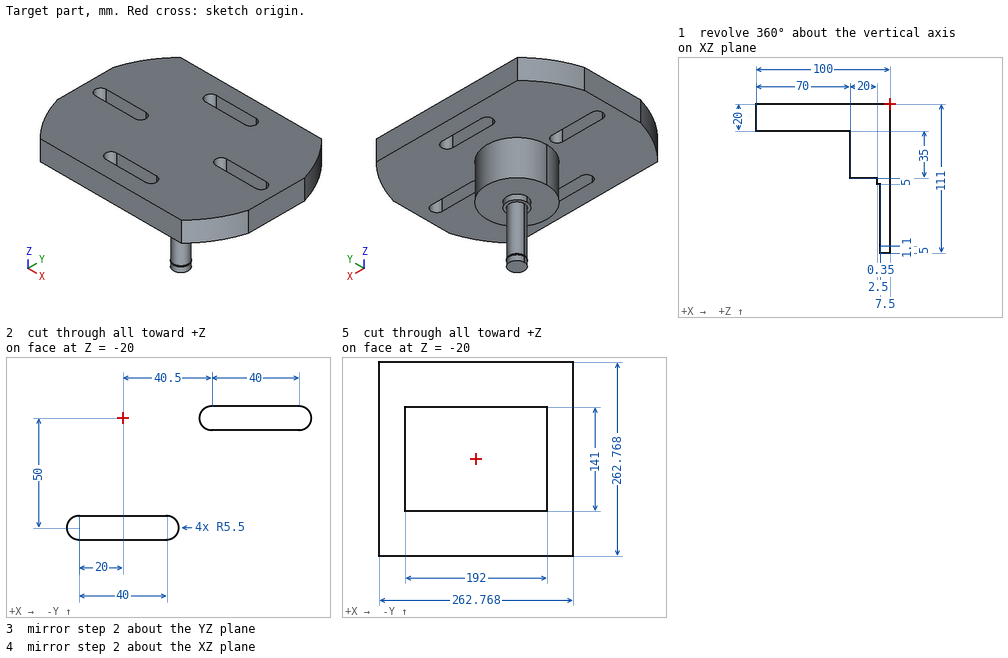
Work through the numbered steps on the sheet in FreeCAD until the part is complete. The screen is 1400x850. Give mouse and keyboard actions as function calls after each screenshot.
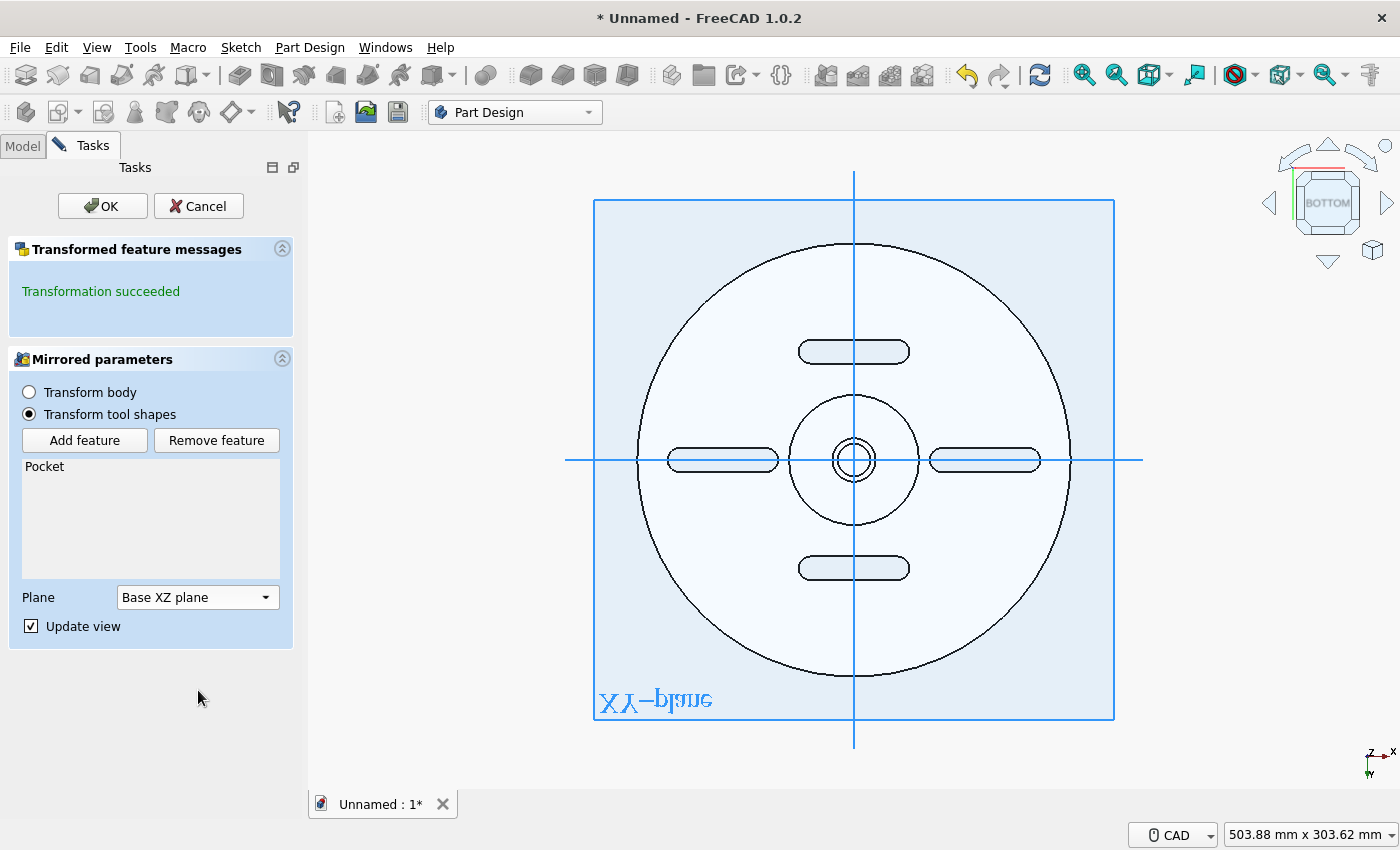
click(103, 206)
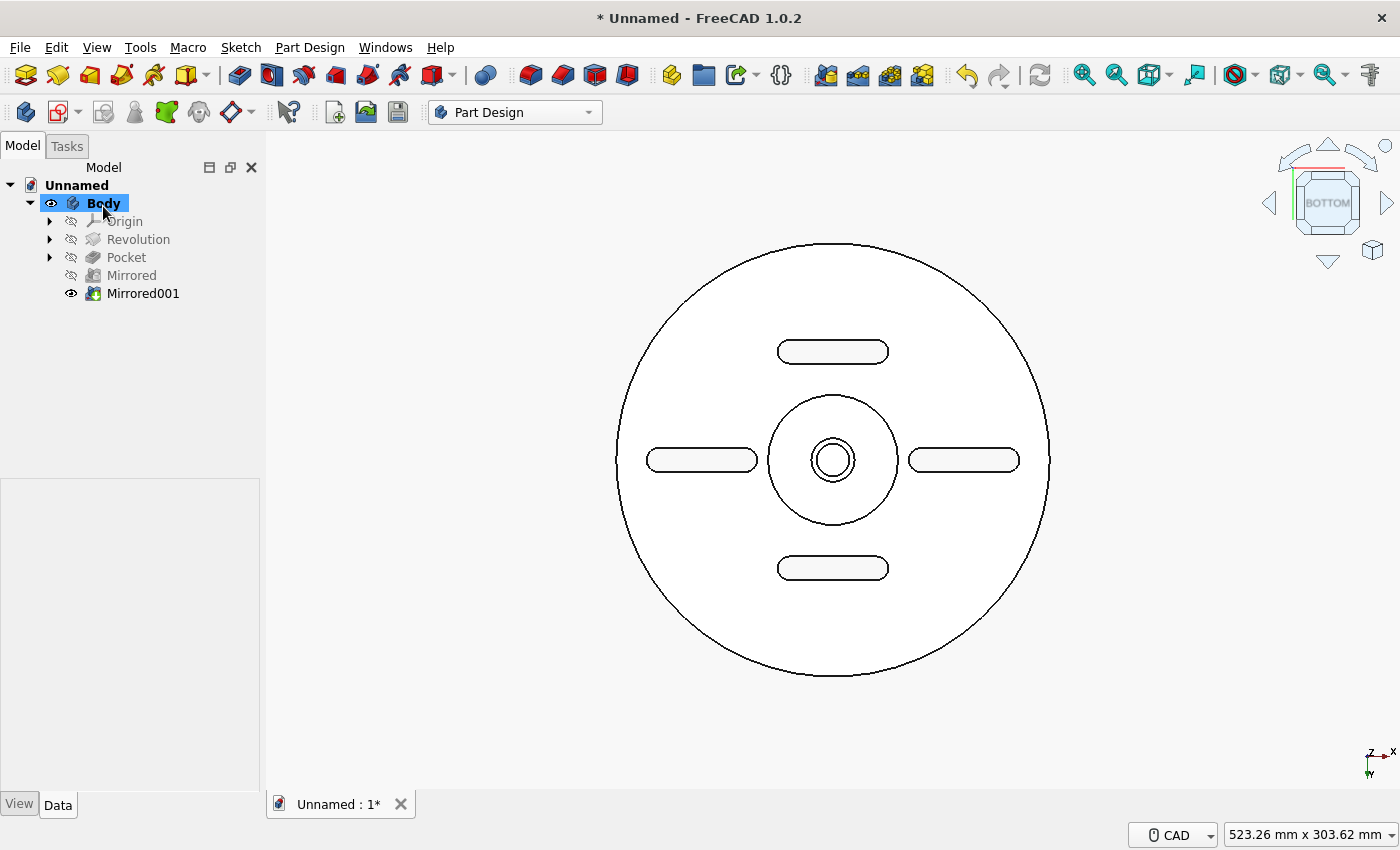
click(709, 397)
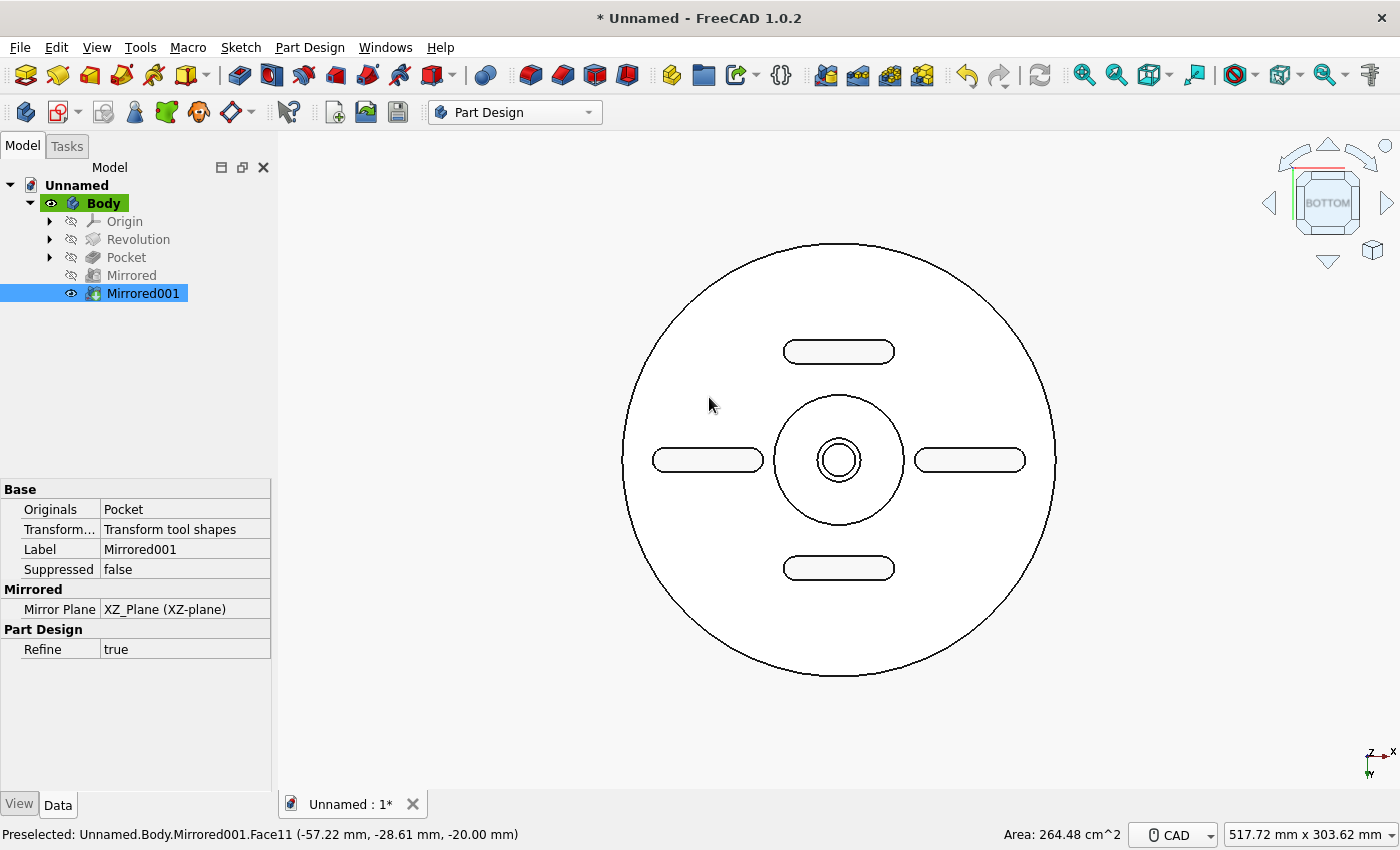
click(58, 112)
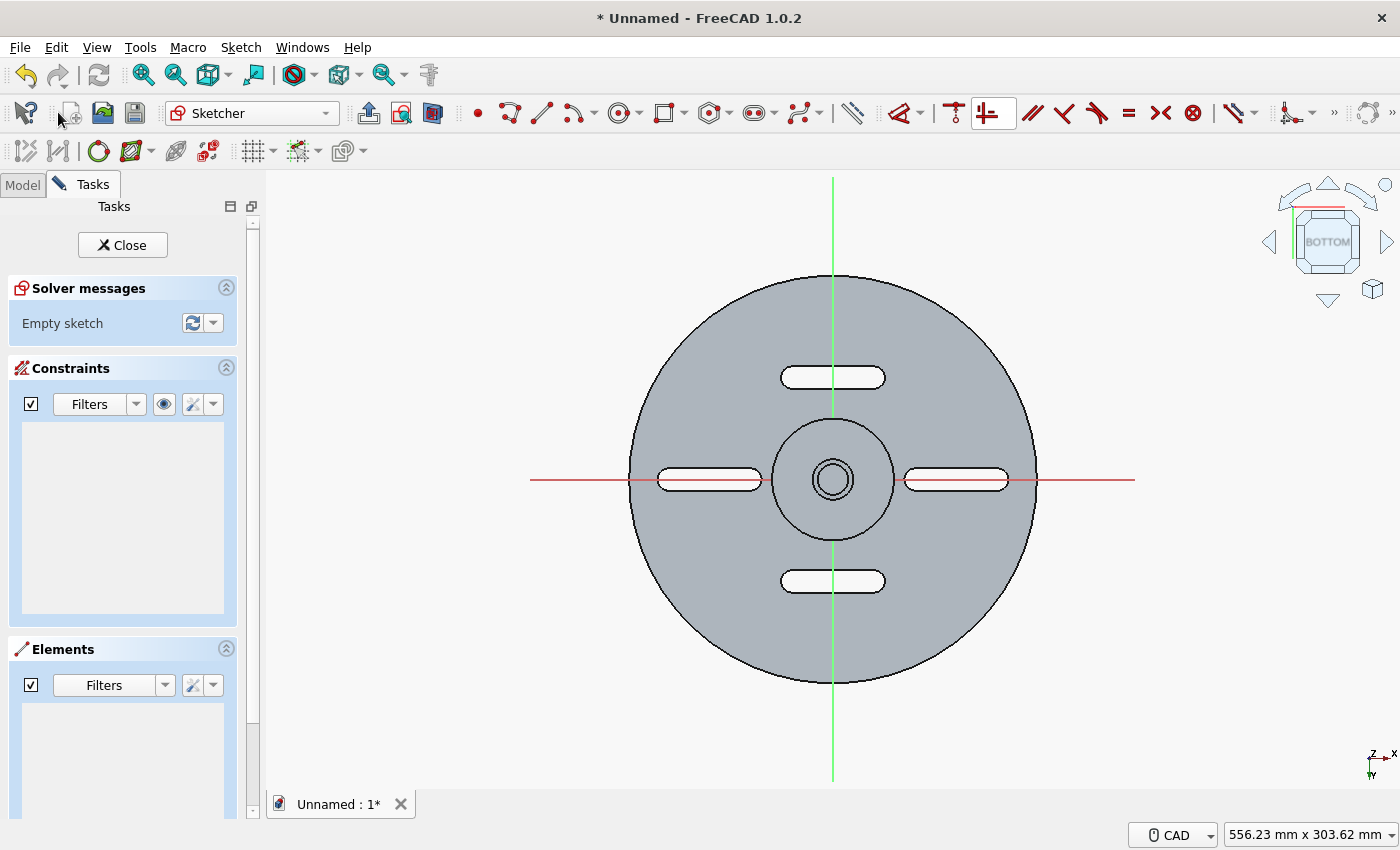
scroll(455, 479, down, 1)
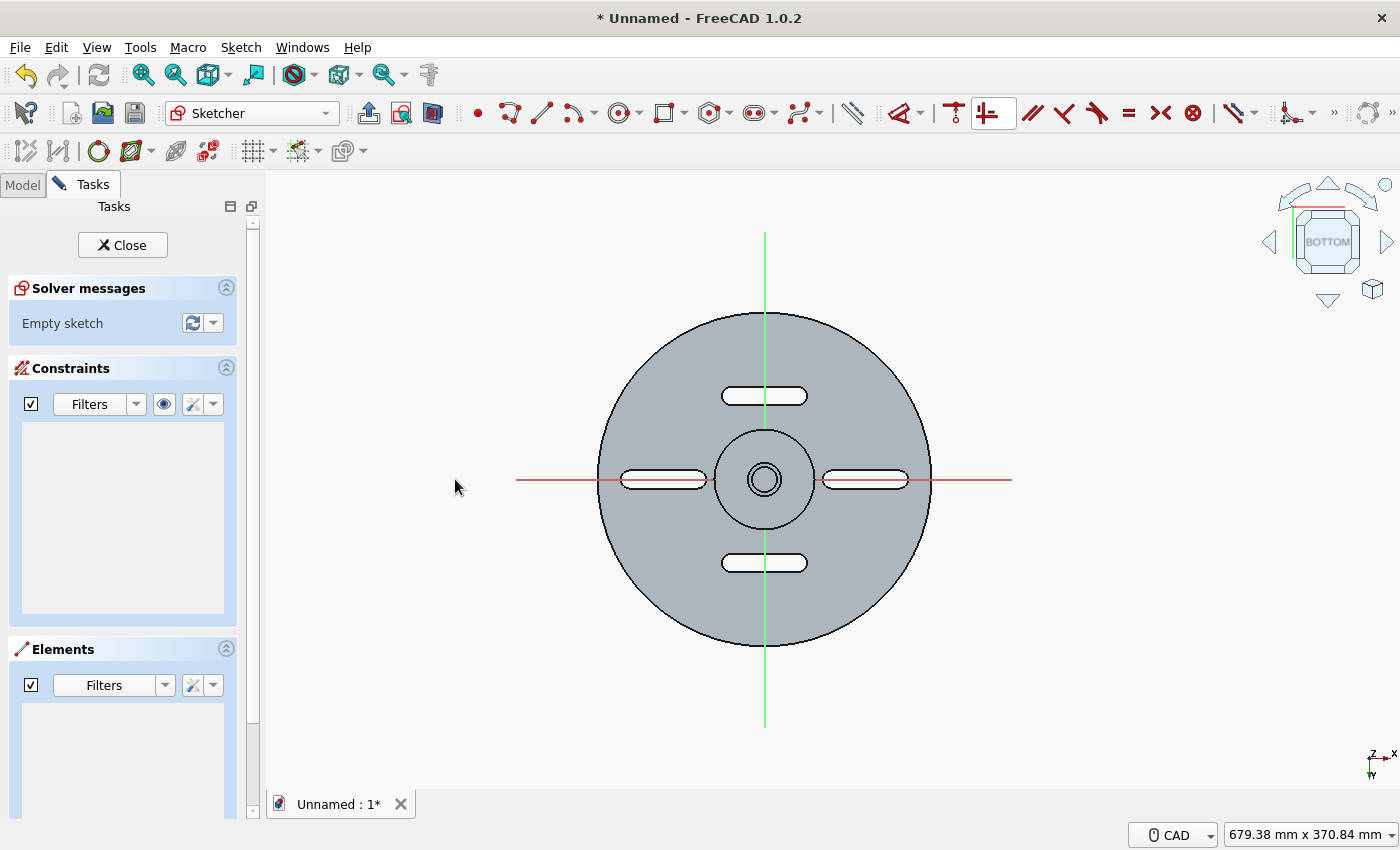
click(686, 114)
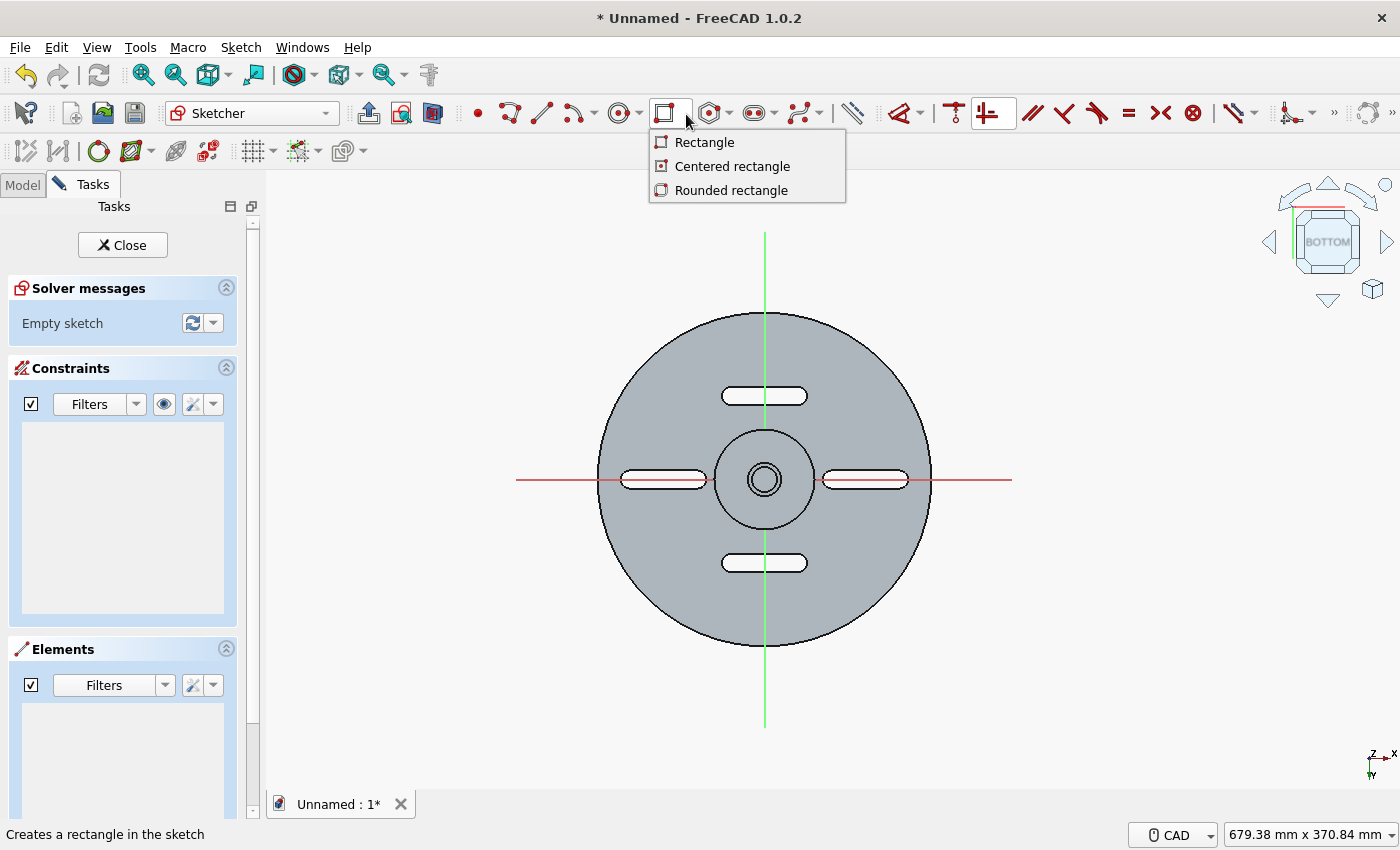
click(748, 166)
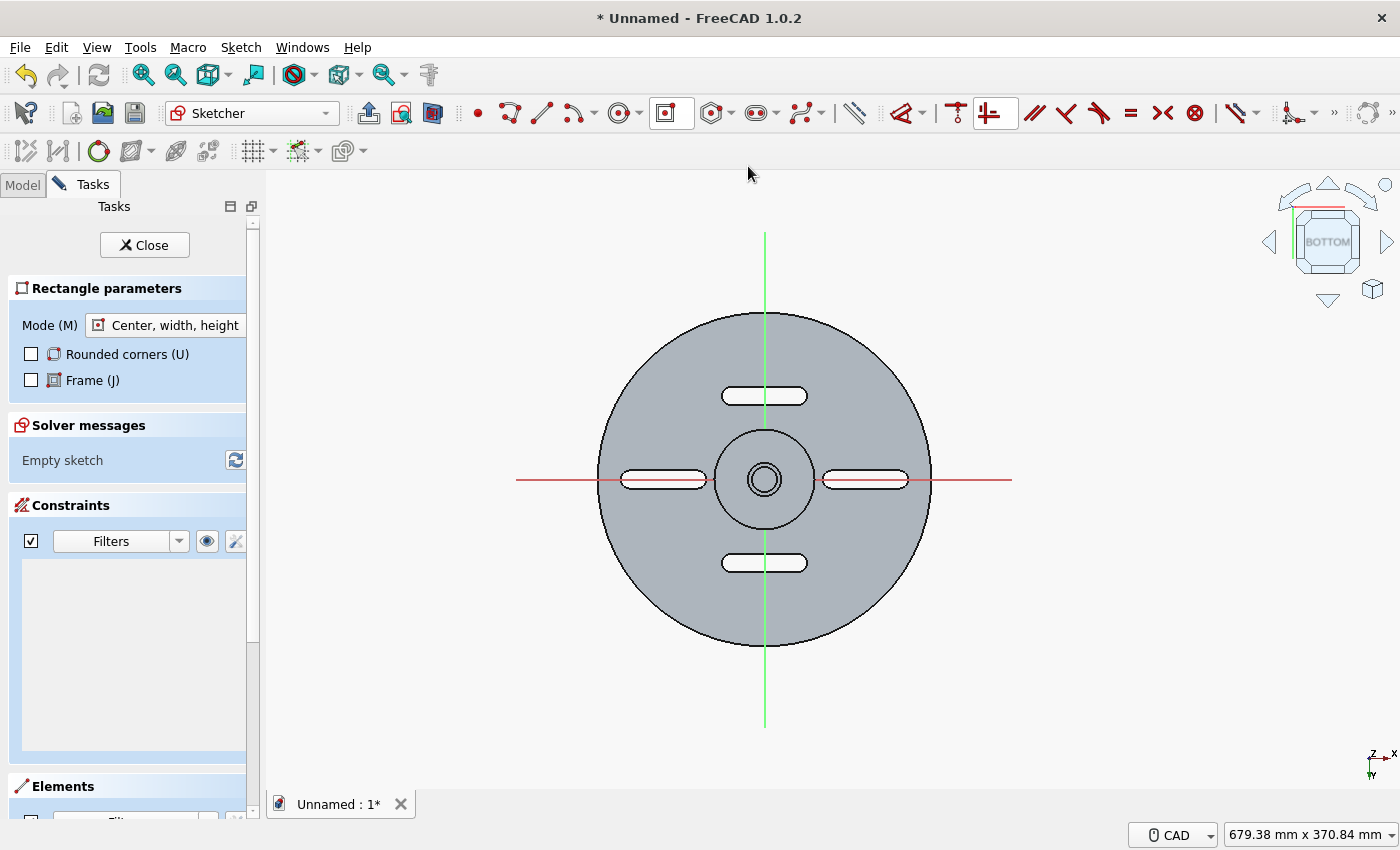
click(765, 480)
click(984, 260)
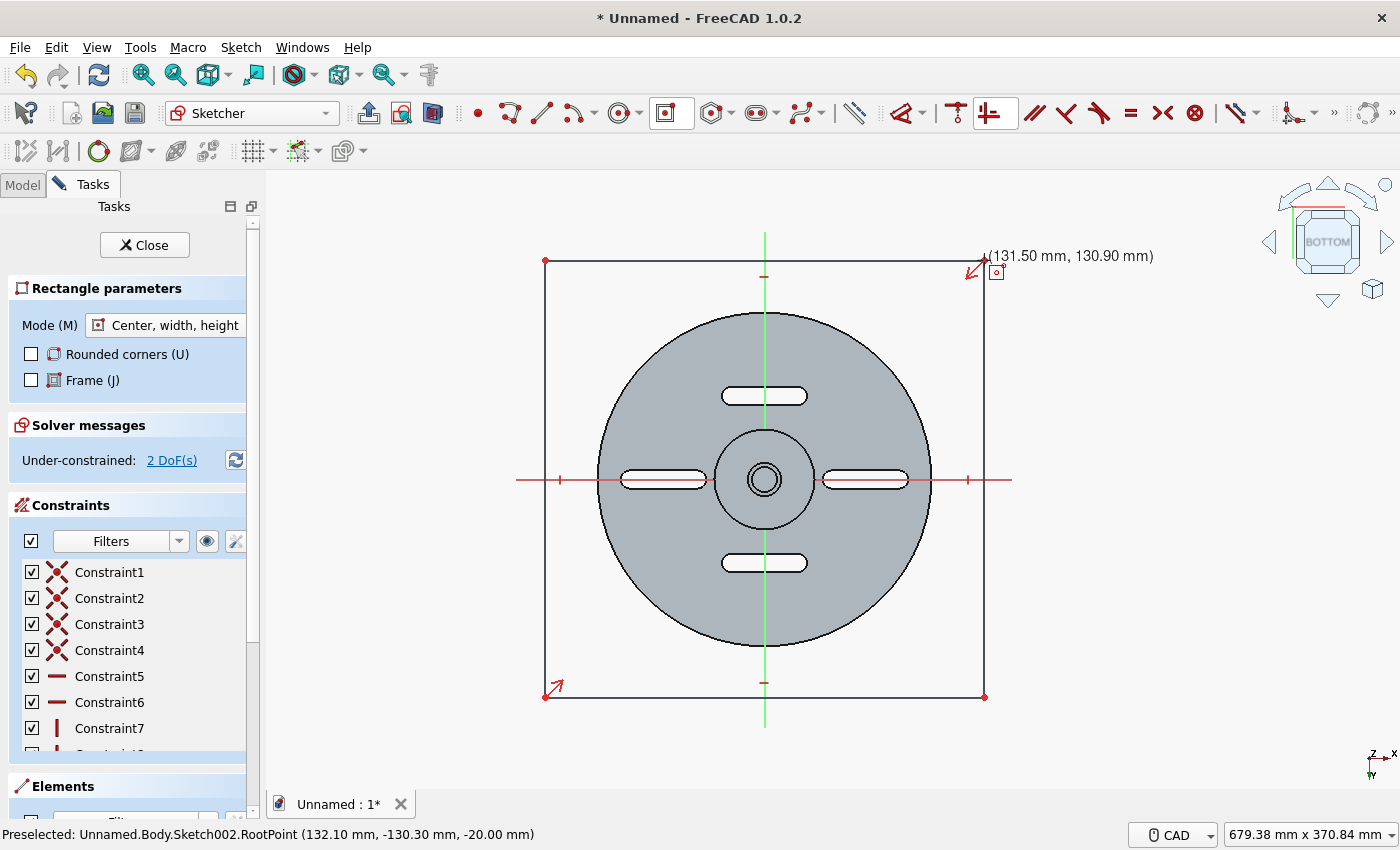
click(765, 480)
click(925, 362)
key(Escape)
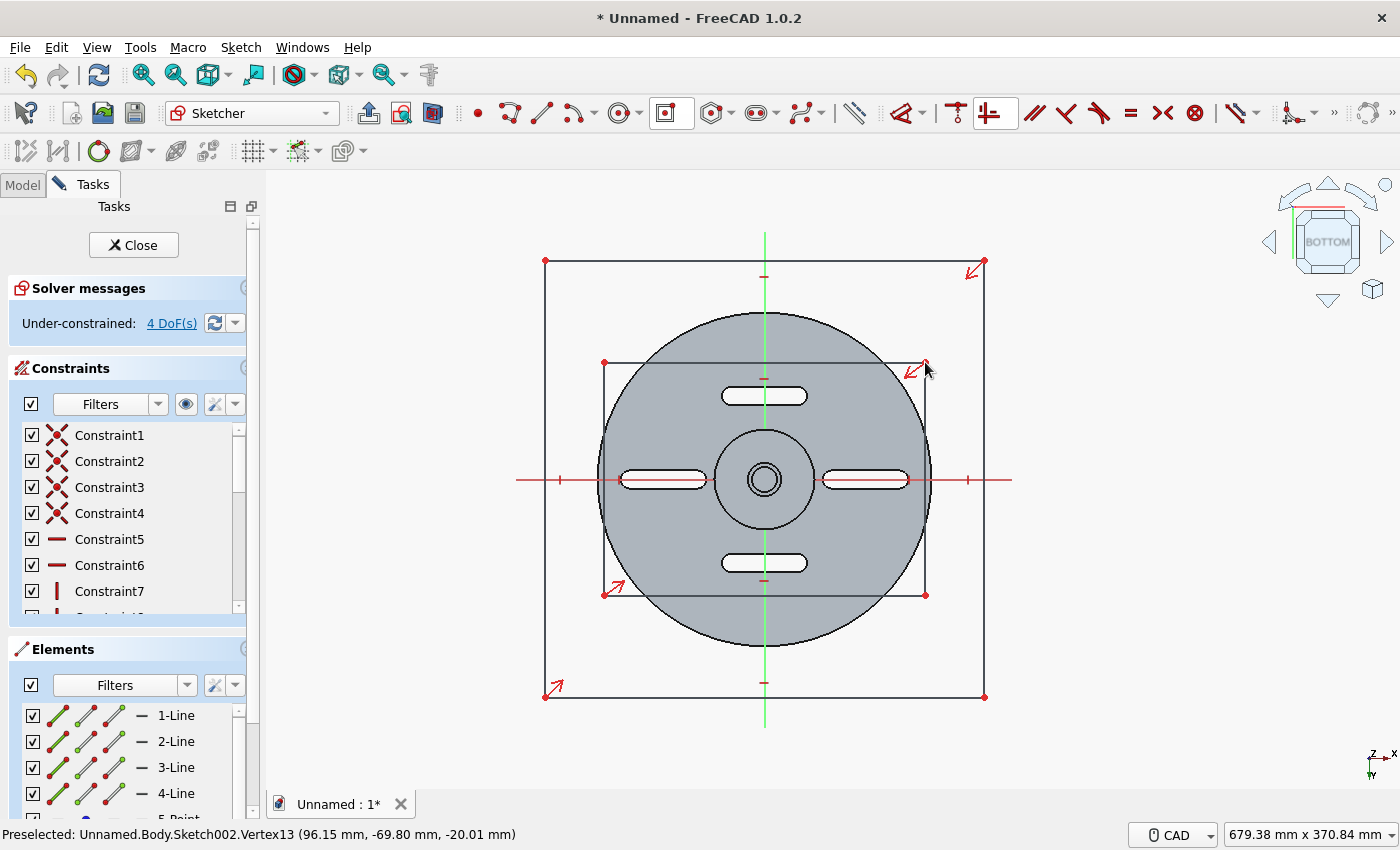
click(902, 114)